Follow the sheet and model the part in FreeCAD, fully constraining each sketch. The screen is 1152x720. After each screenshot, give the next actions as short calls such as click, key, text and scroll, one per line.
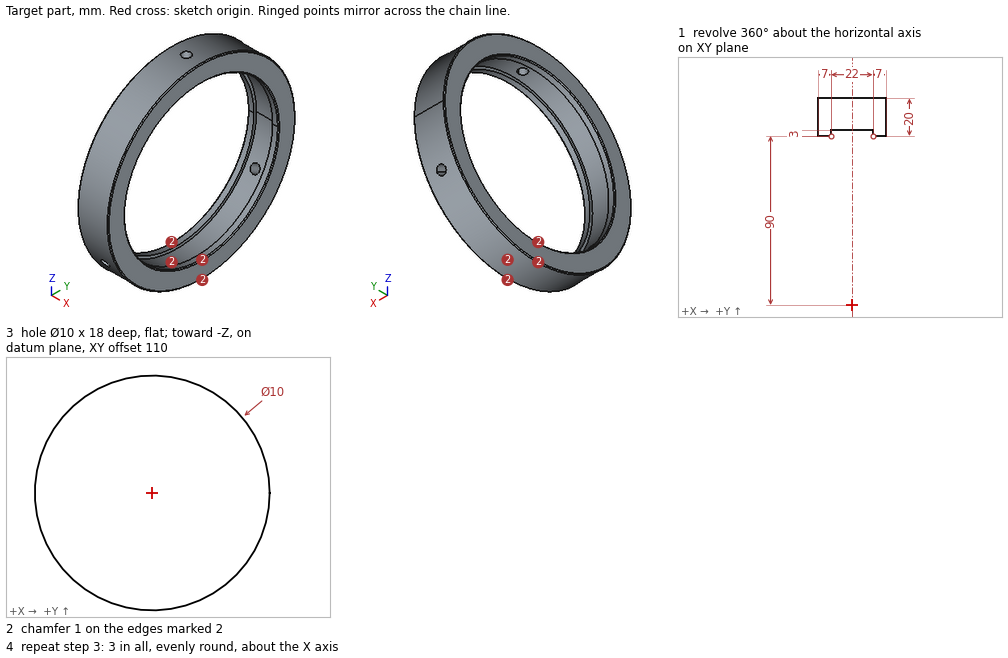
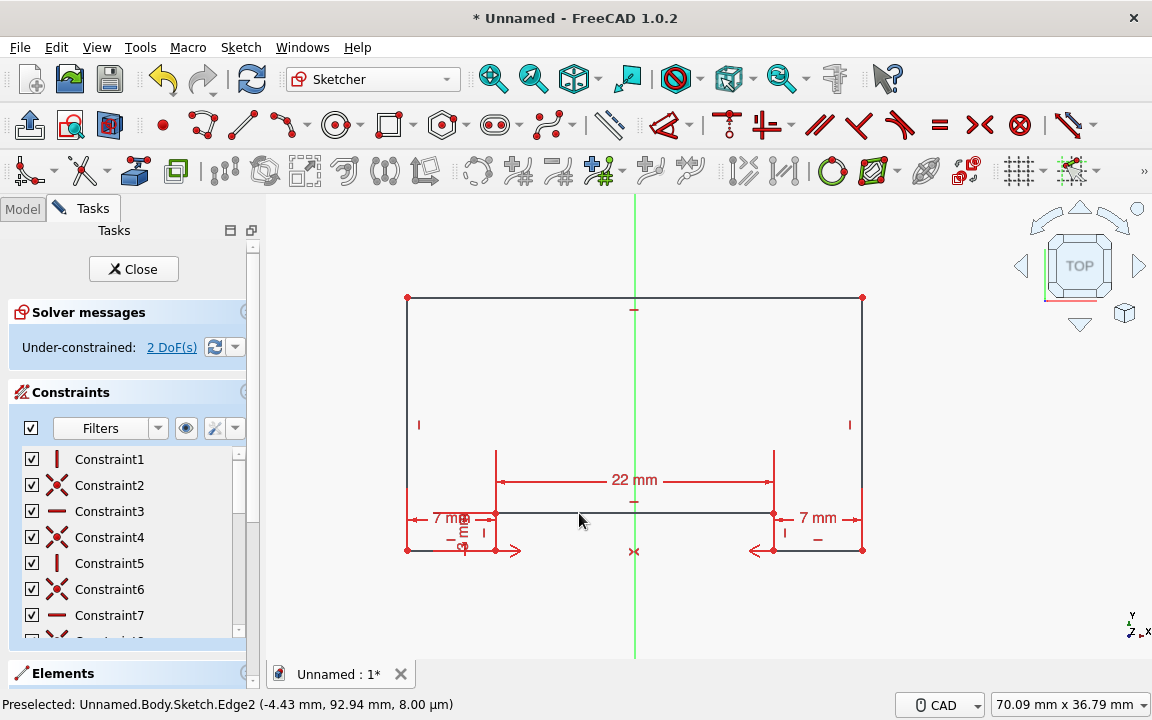
click(862, 475)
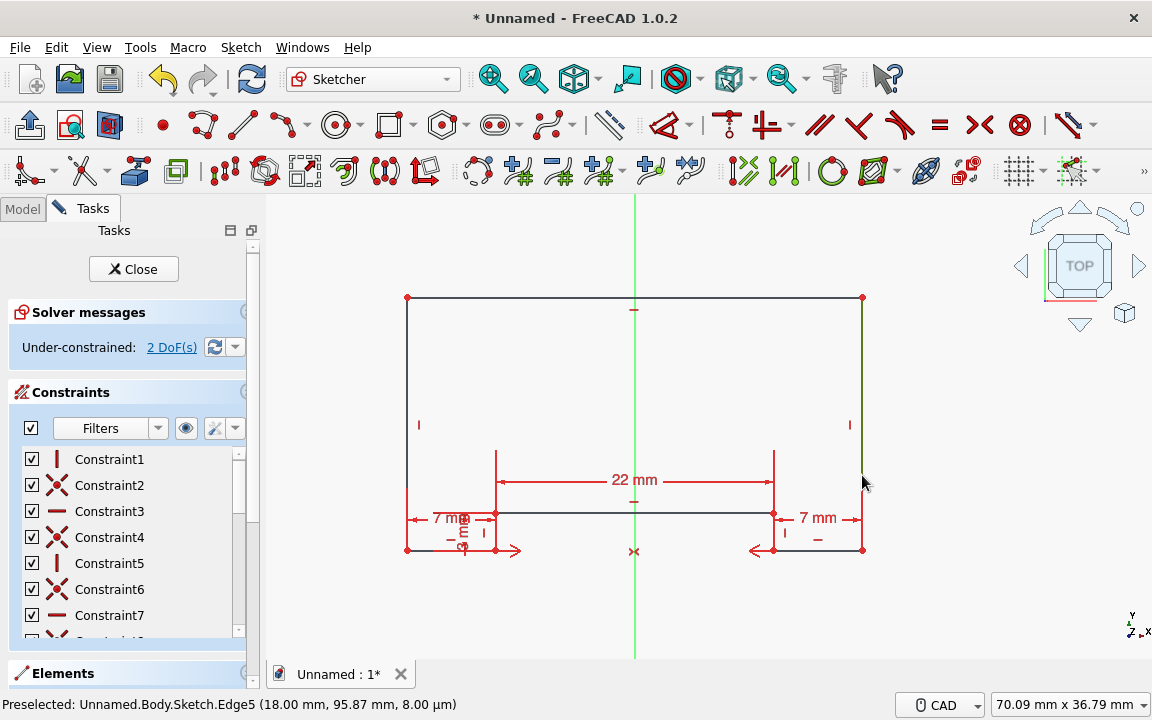
click(692, 126)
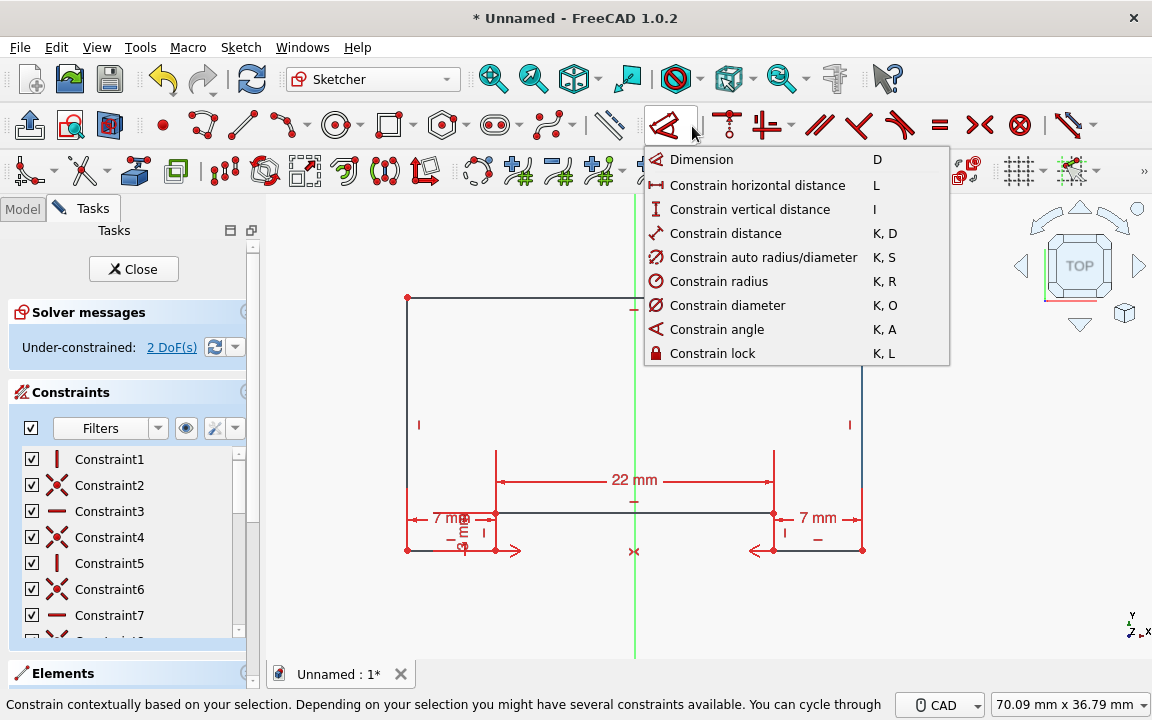
click(797, 209)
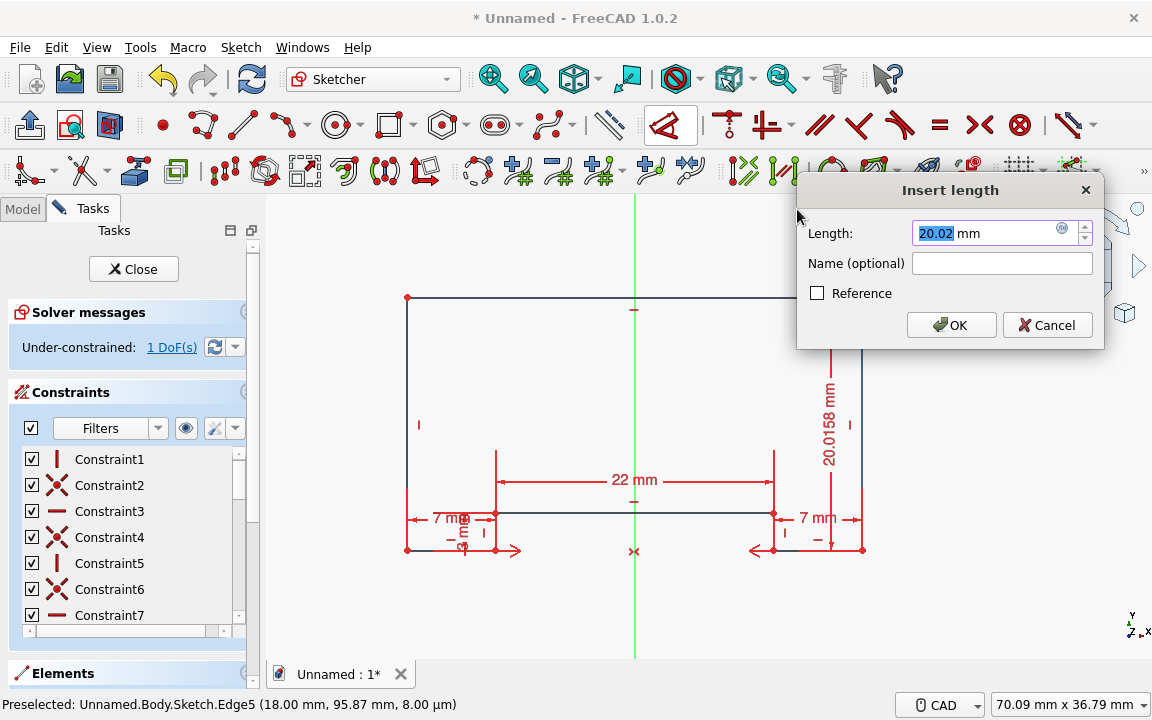
text(20)
key(Return)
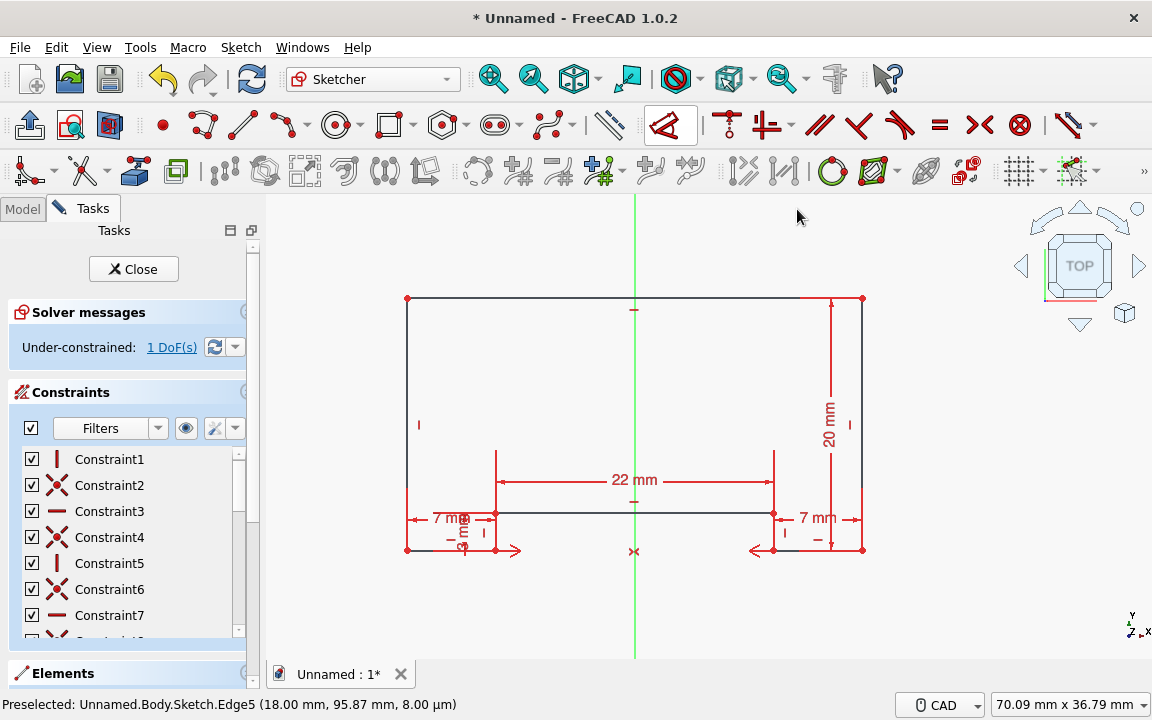
click(496, 551)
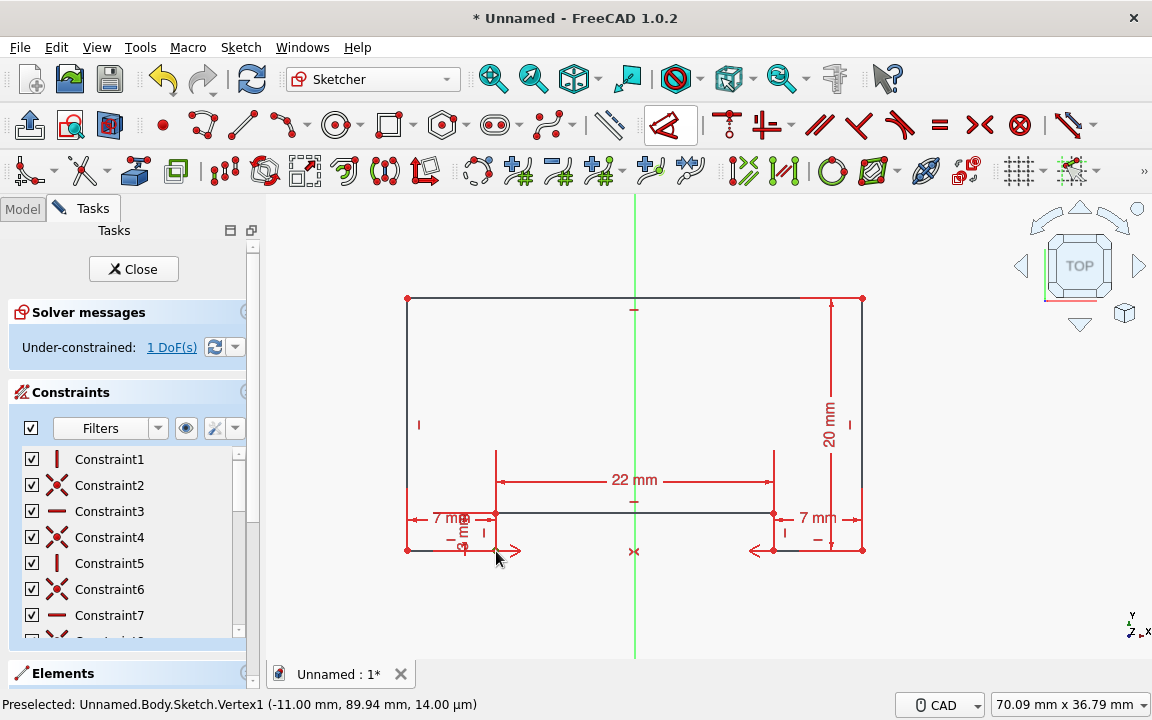
click(692, 126)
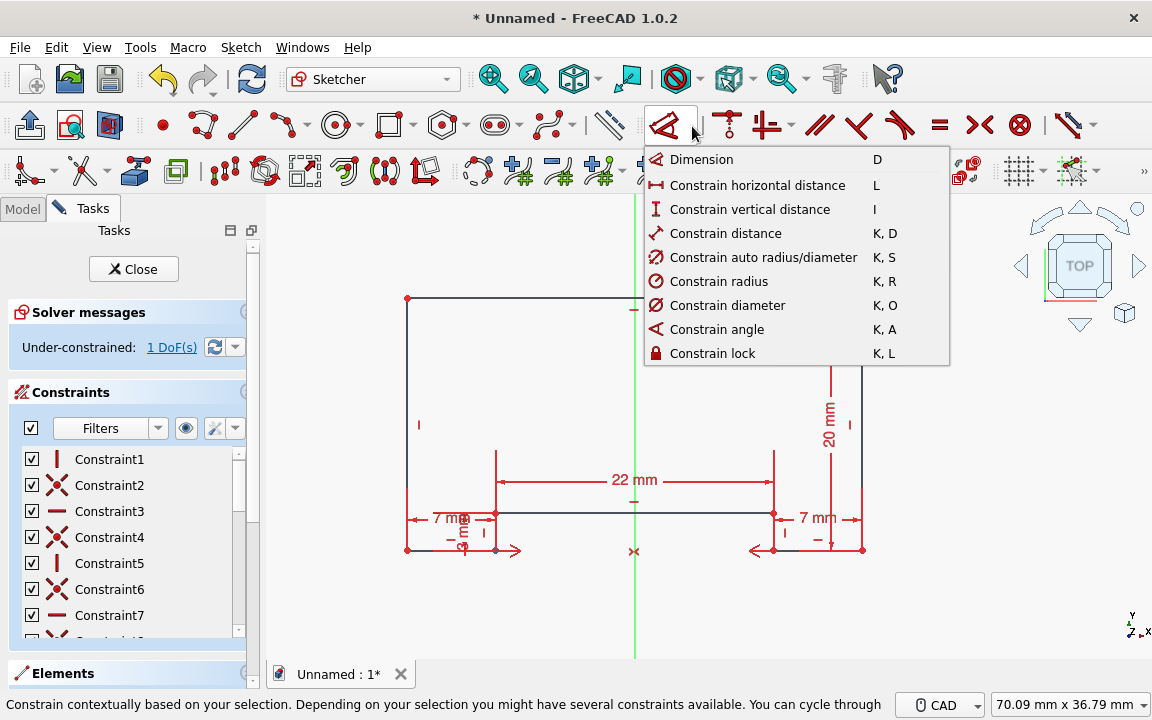
click(797, 209)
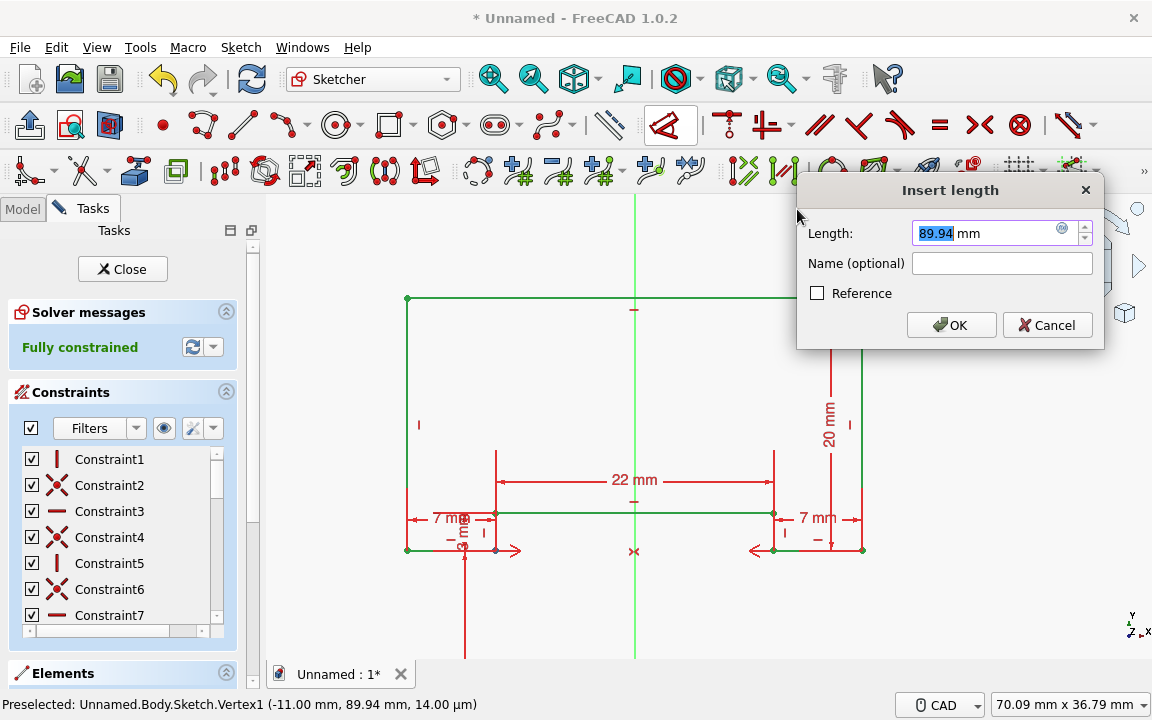
text(90)
key(Return)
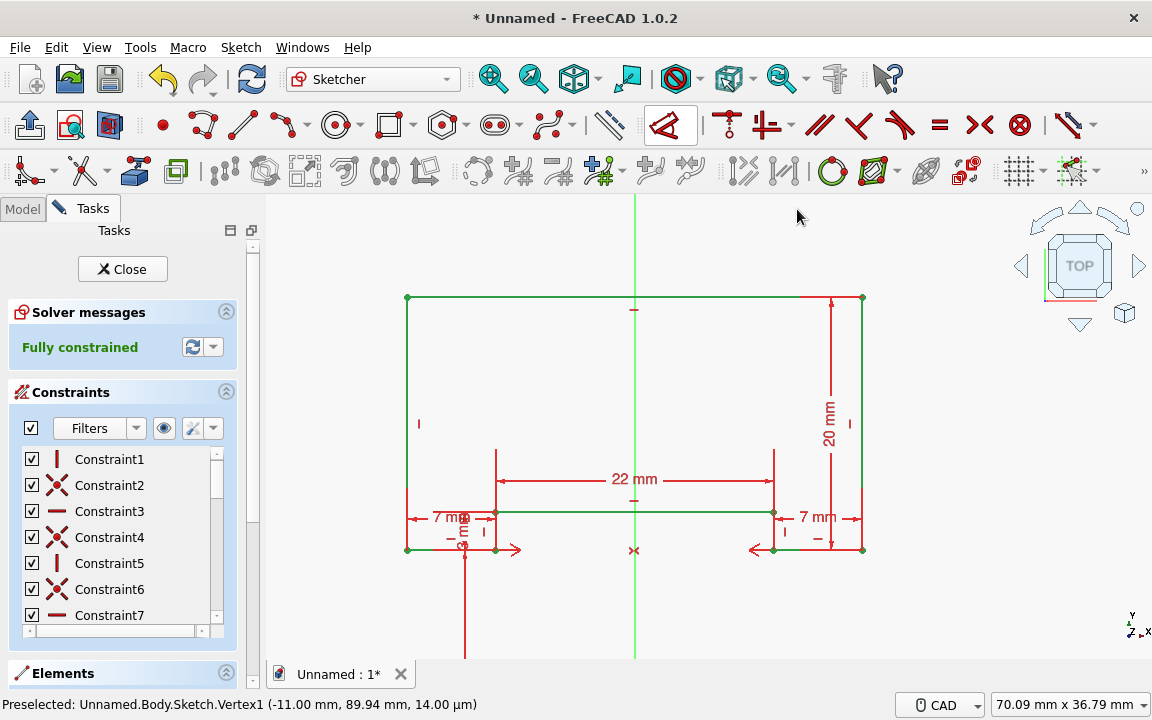
click(123, 269)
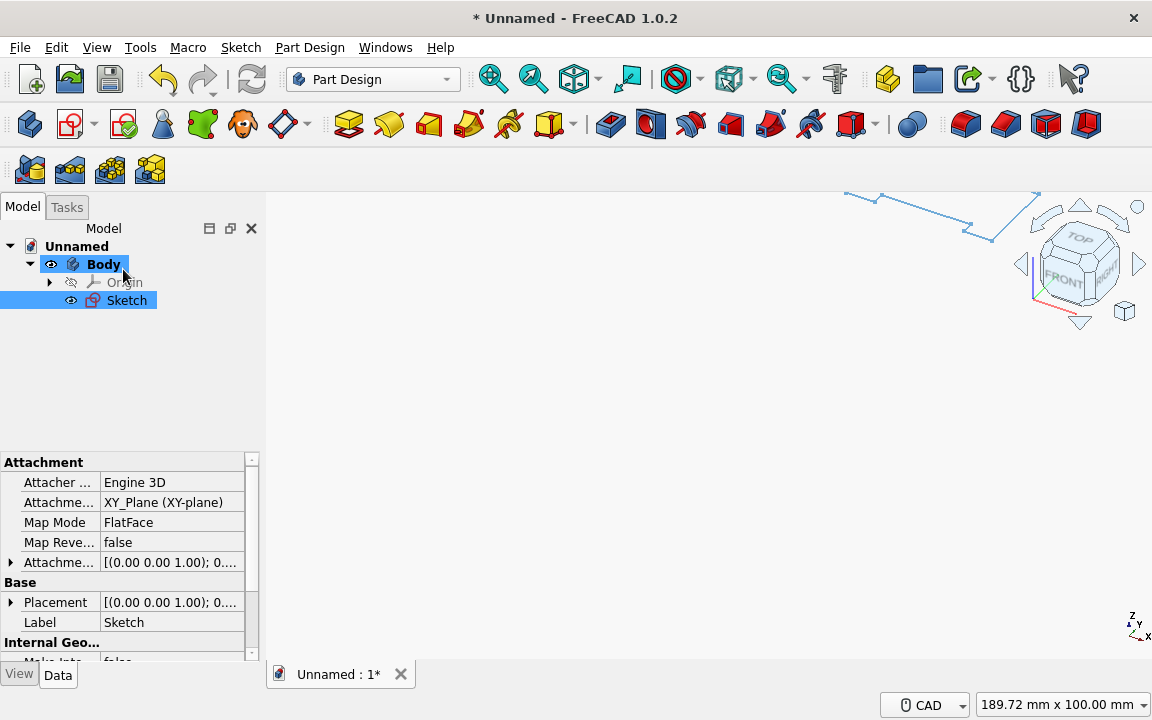
click(390, 124)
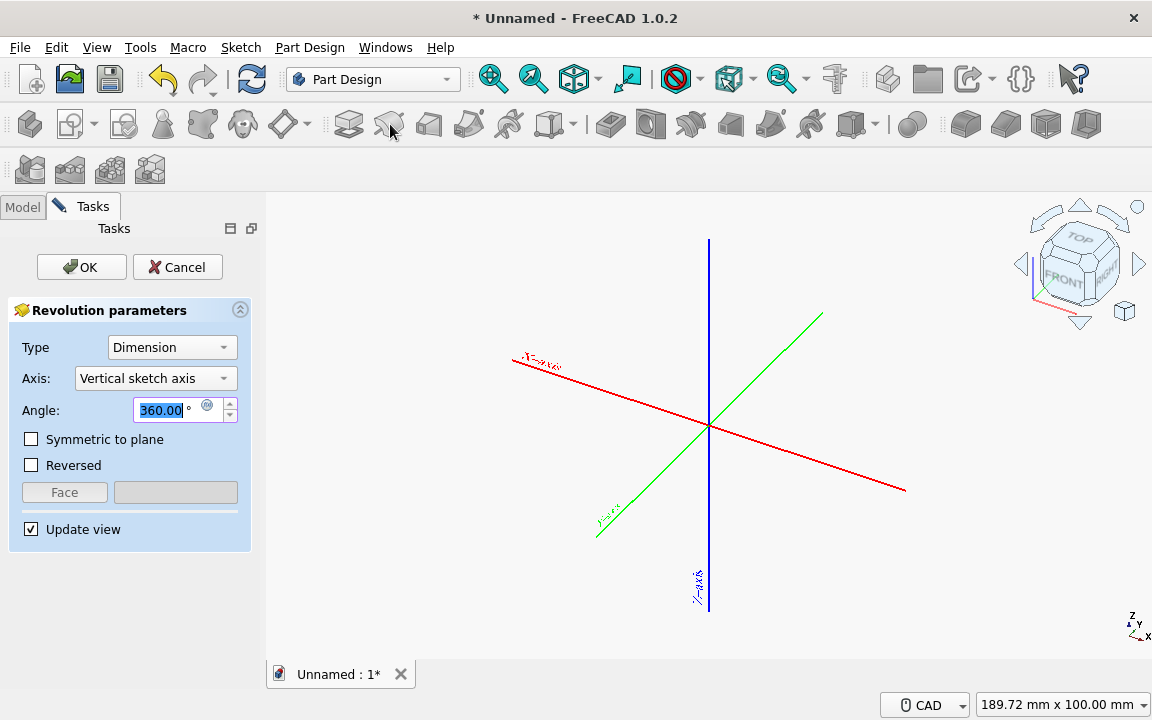
click(156, 378)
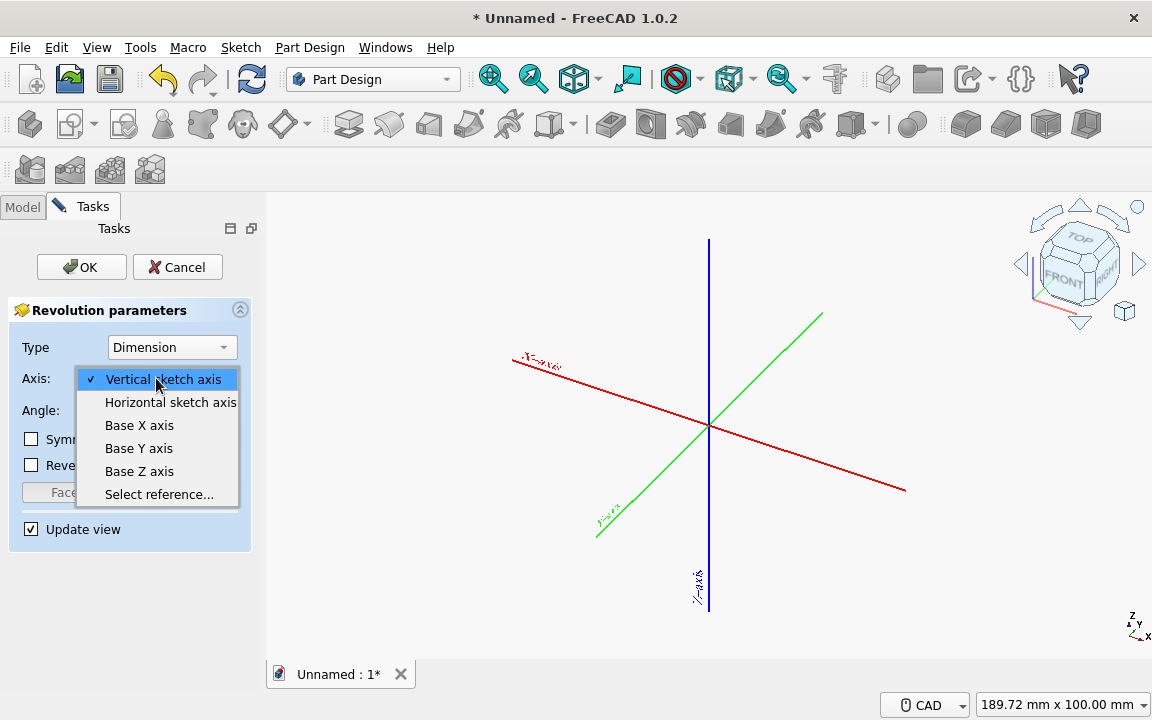
click(156, 402)